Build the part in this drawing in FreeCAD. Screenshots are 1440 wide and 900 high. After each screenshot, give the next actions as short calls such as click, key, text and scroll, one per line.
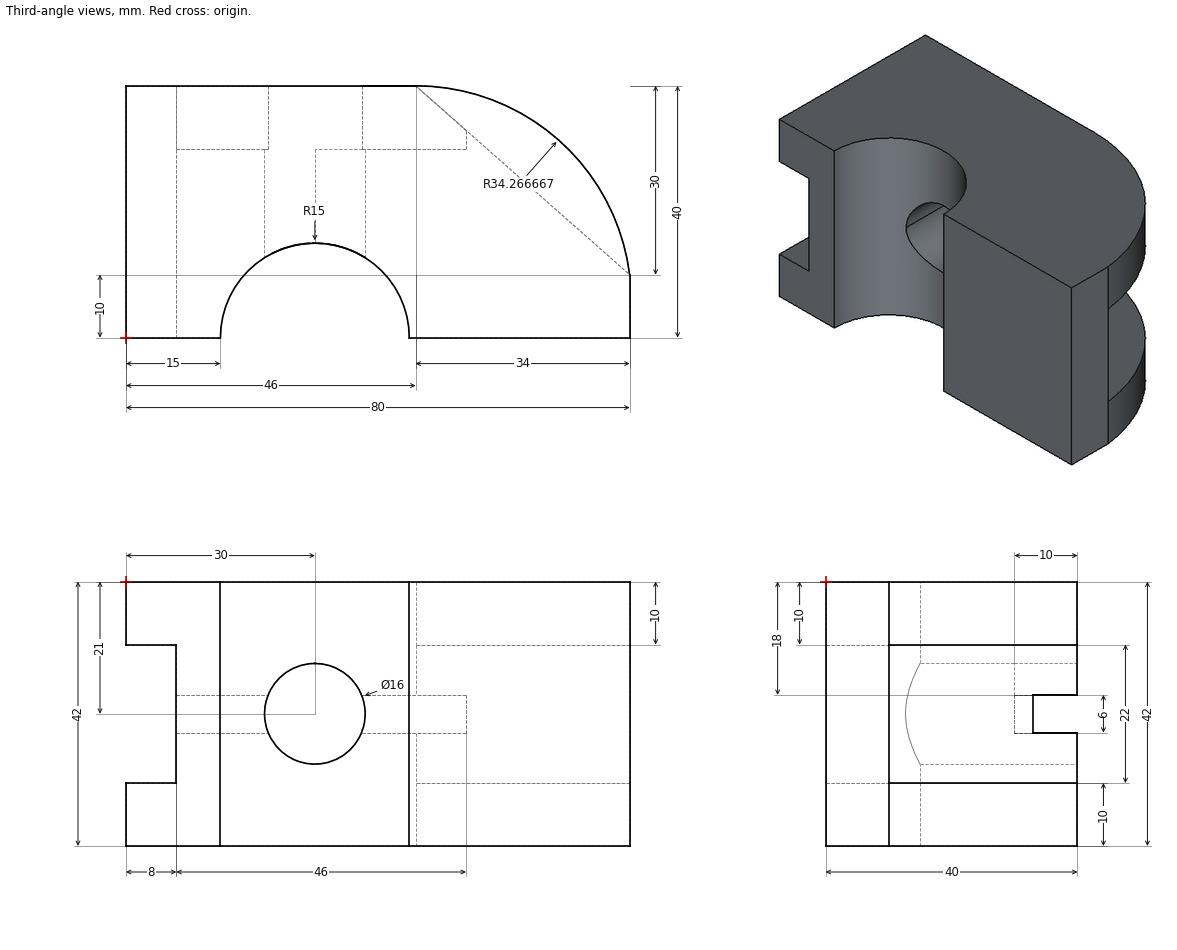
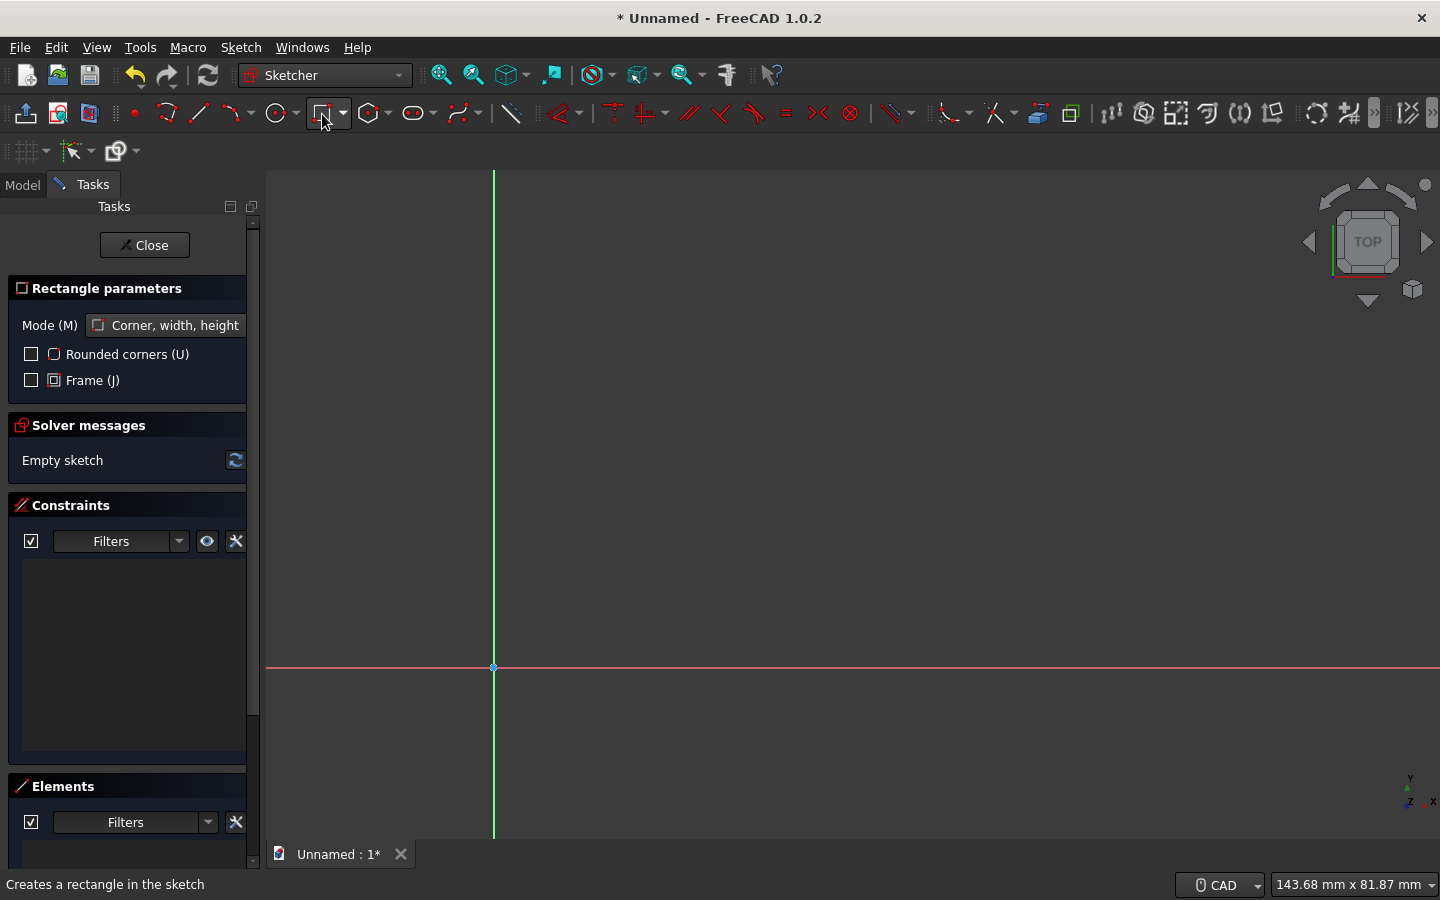
click(494, 668)
move(1148, 341)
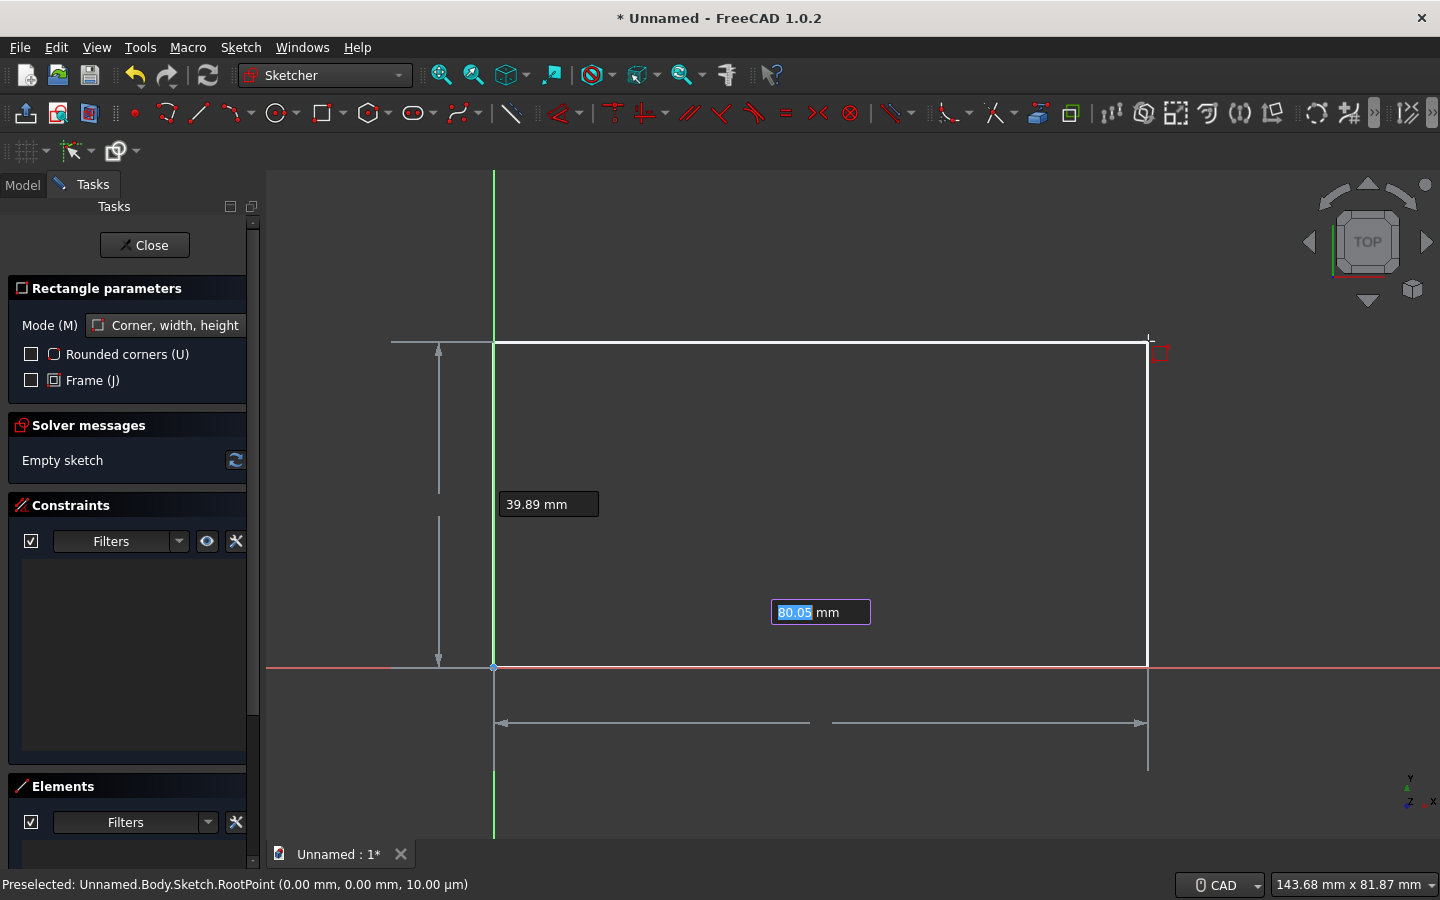
text(80)
key(Tab)
text(40)
key(Return)
key(Escape)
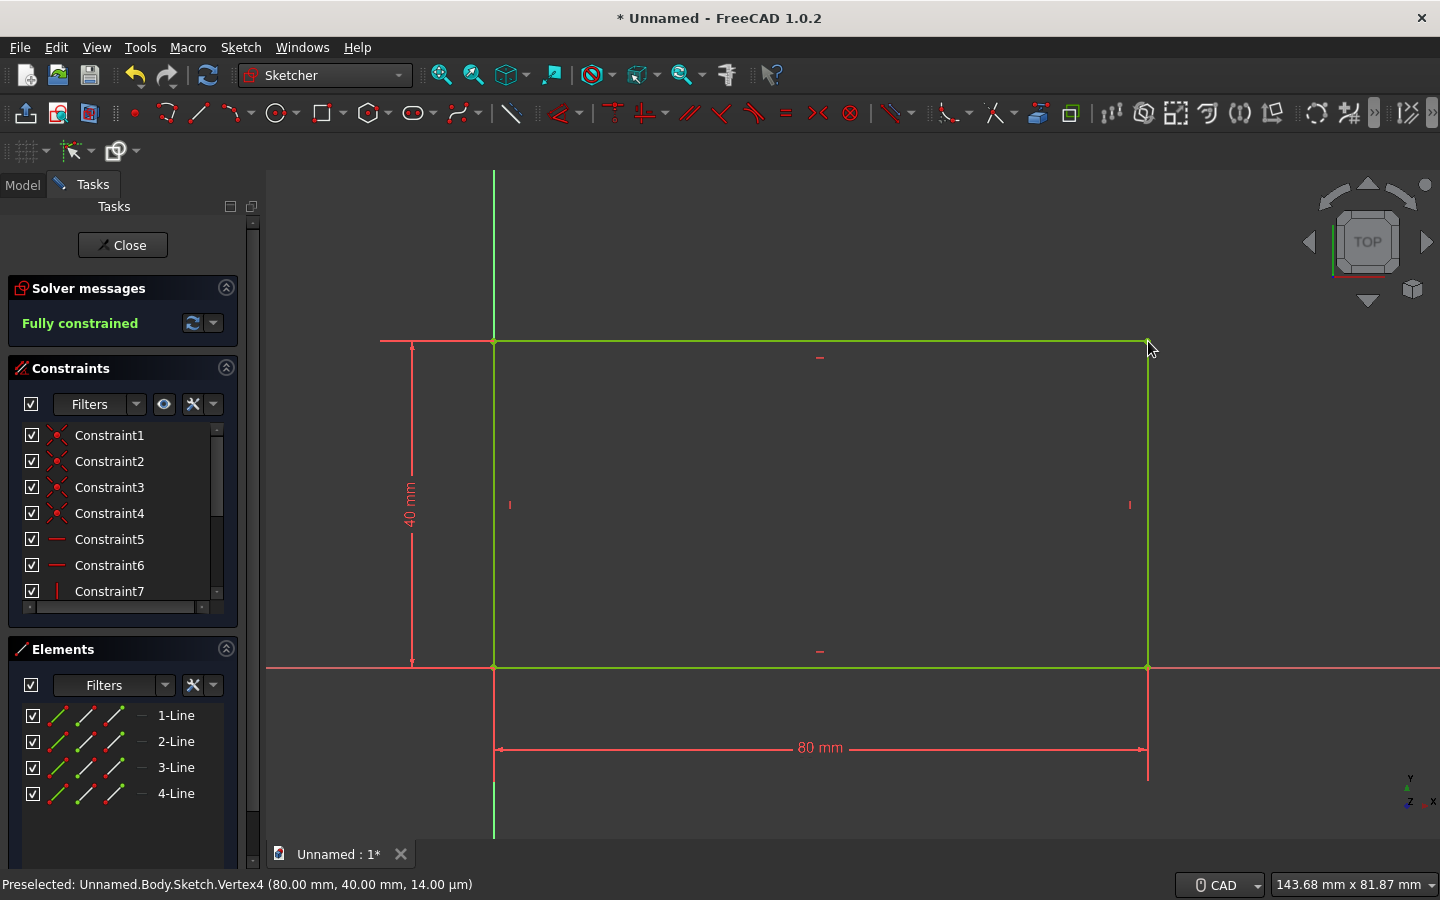
click(123, 245)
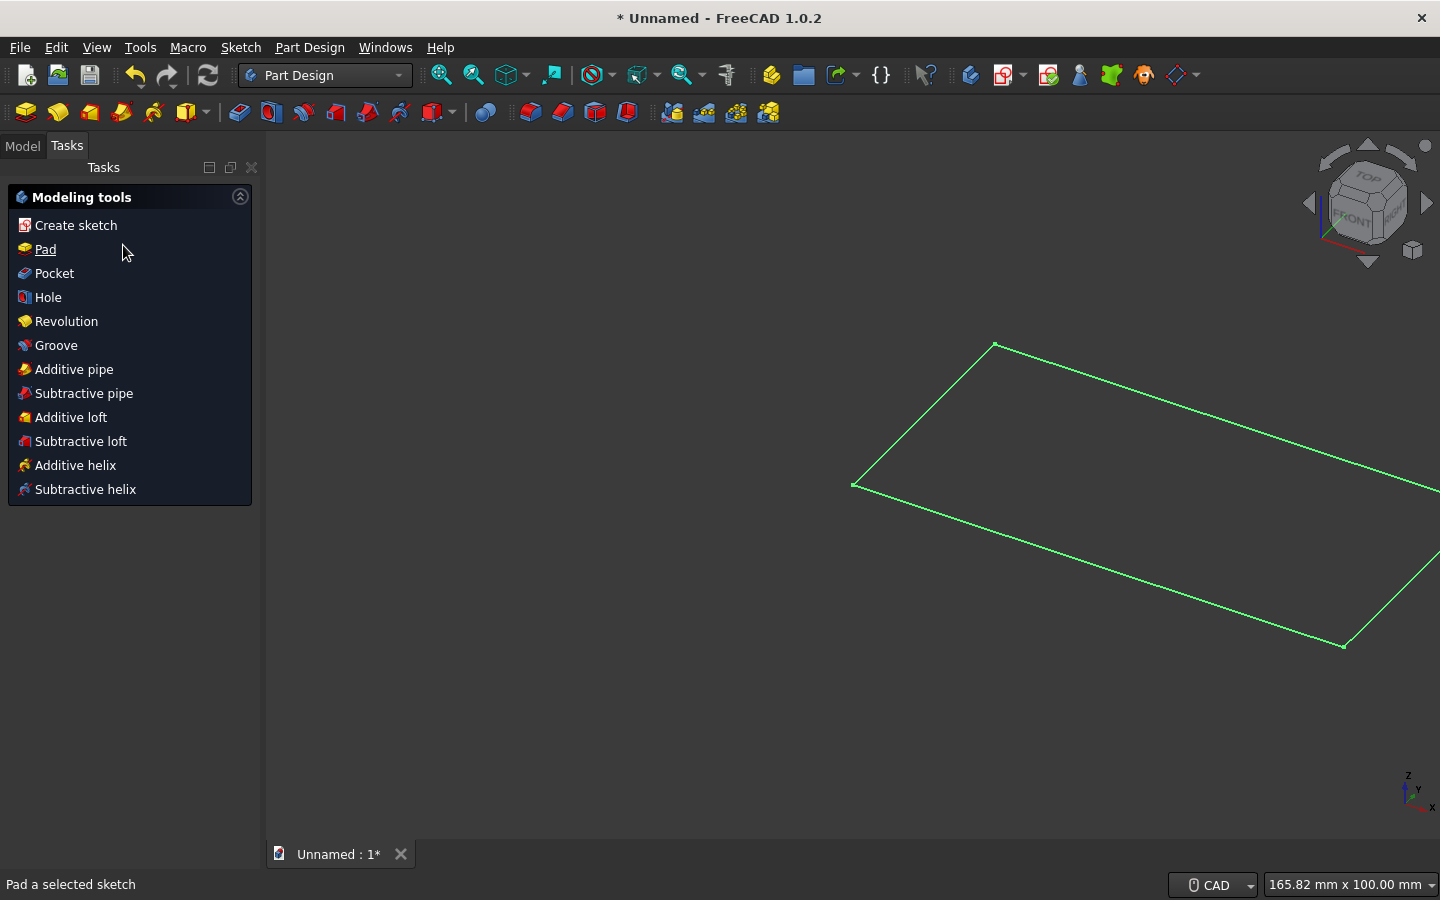
click(26, 112)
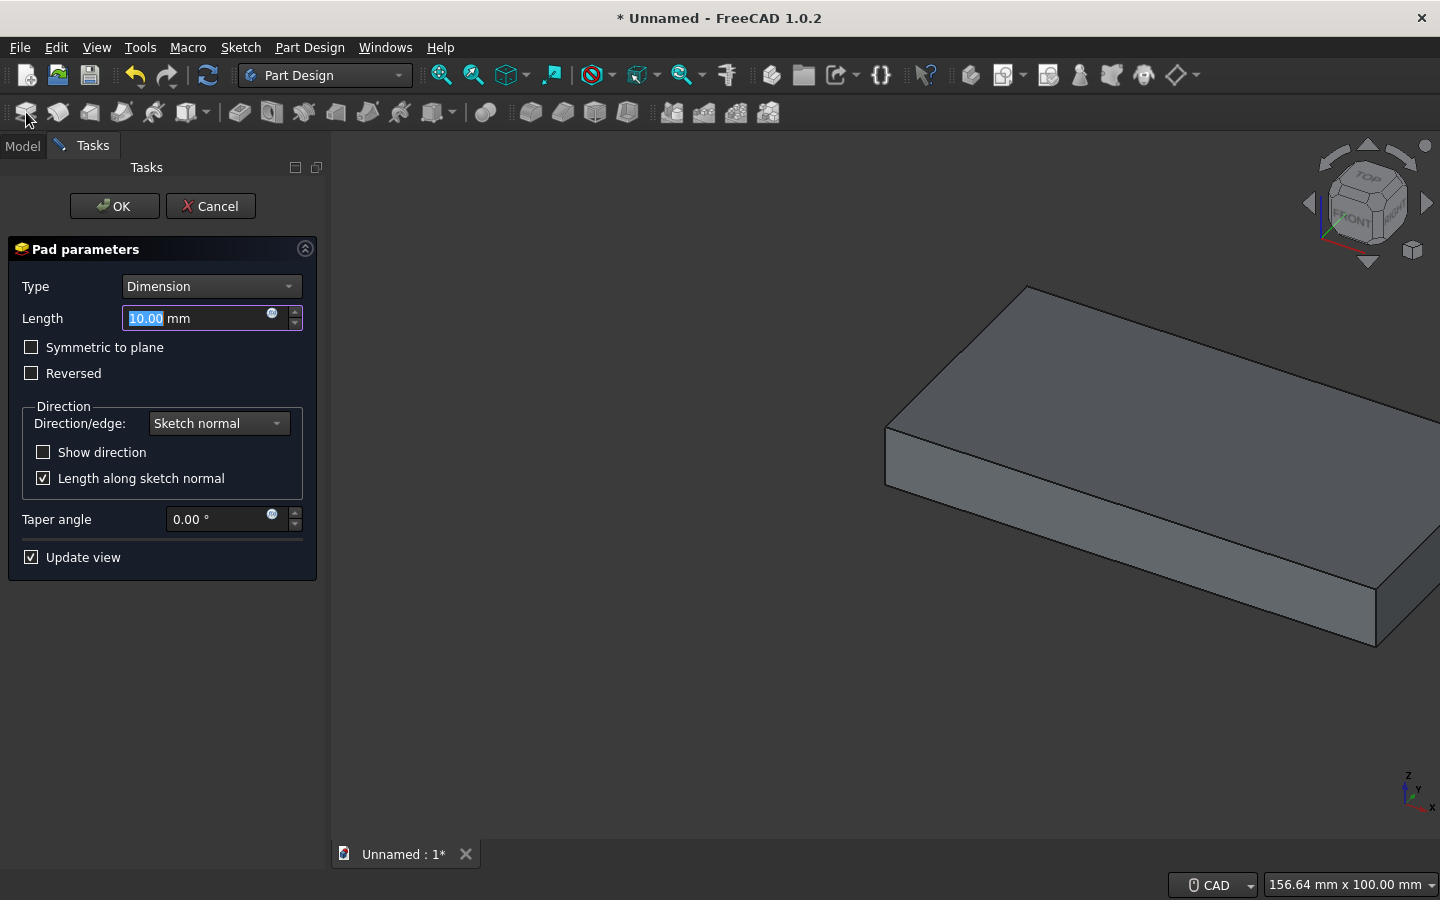
text(42)
key(Tab)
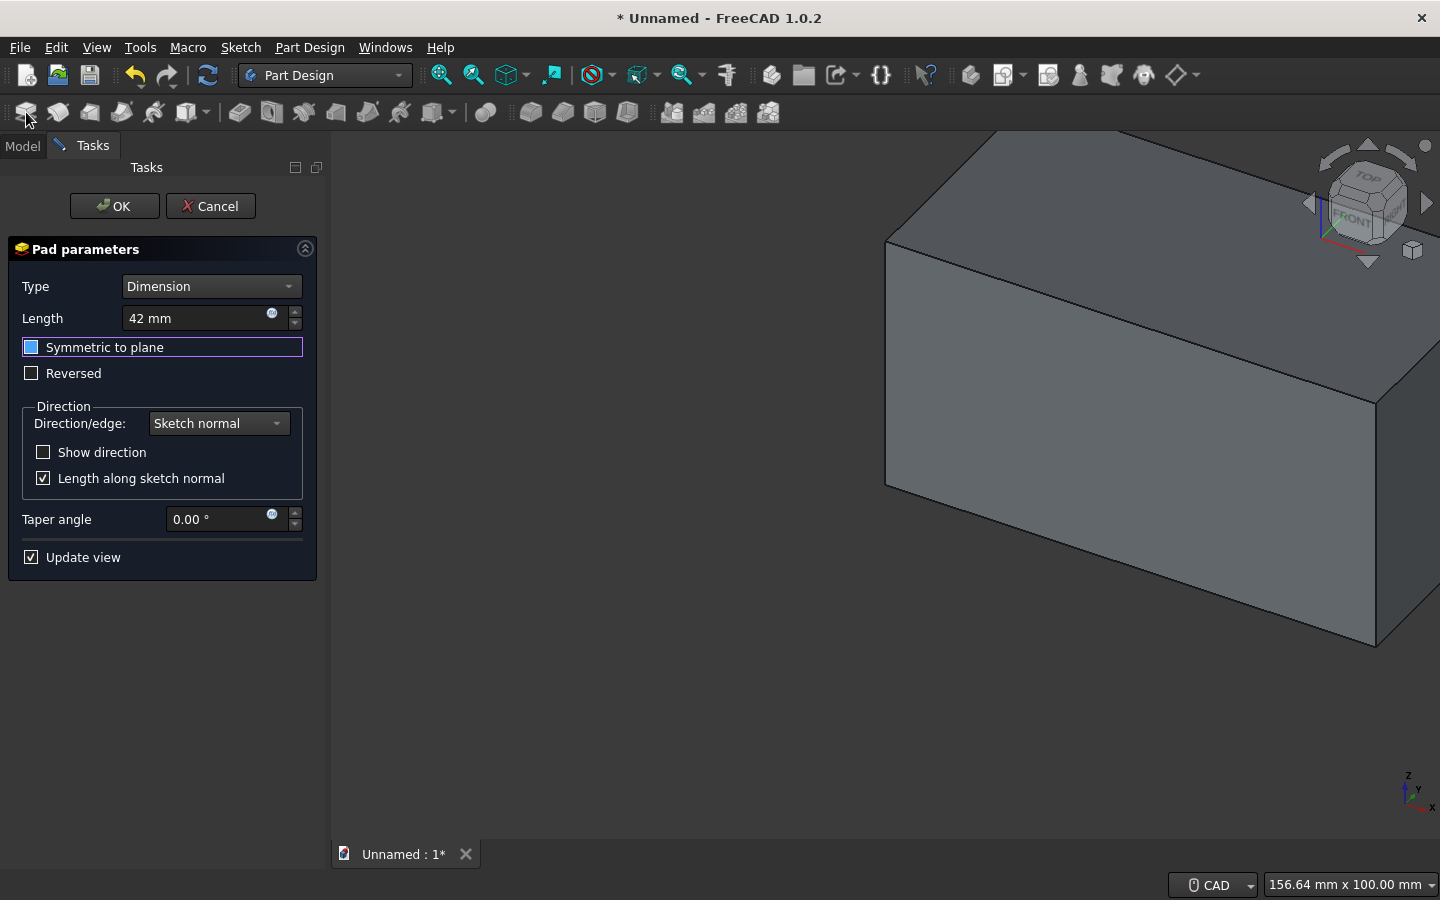
click(30, 373)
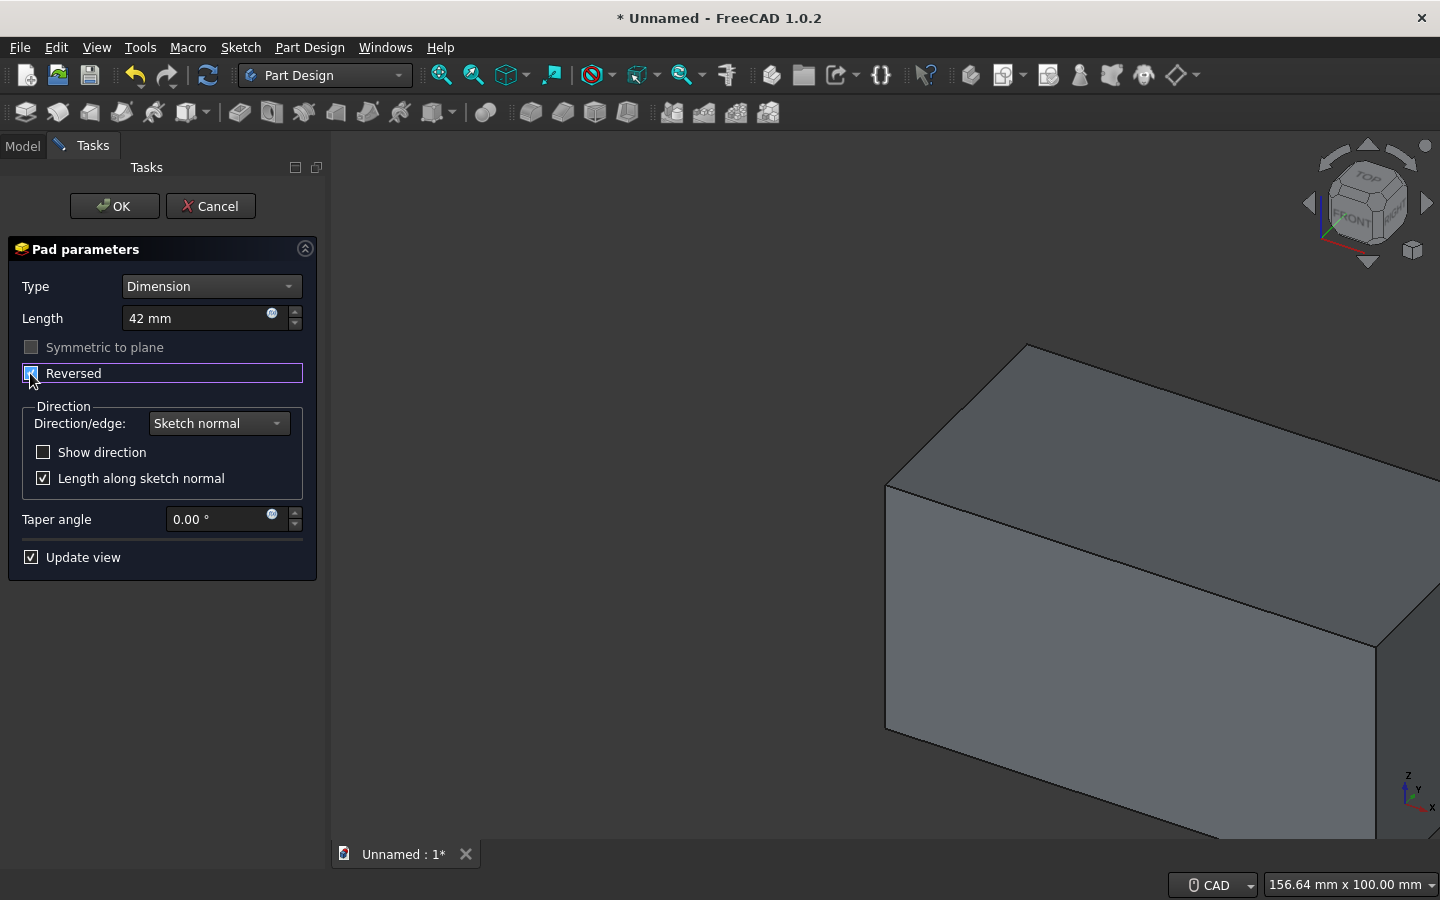
click(115, 206)